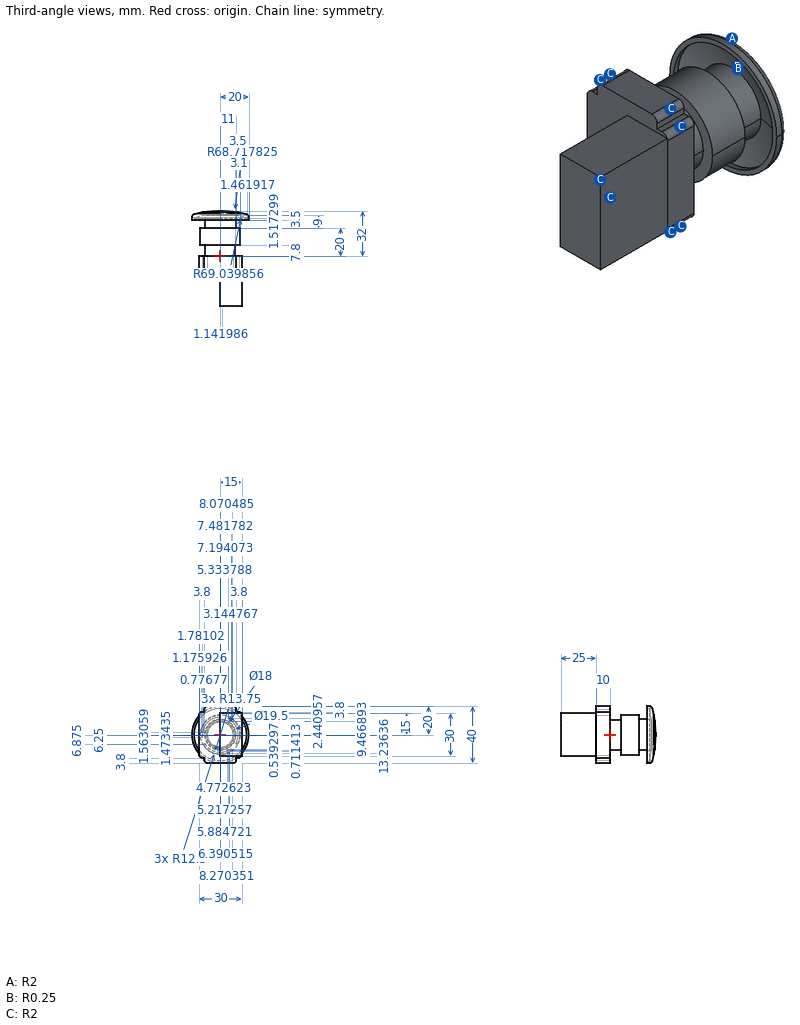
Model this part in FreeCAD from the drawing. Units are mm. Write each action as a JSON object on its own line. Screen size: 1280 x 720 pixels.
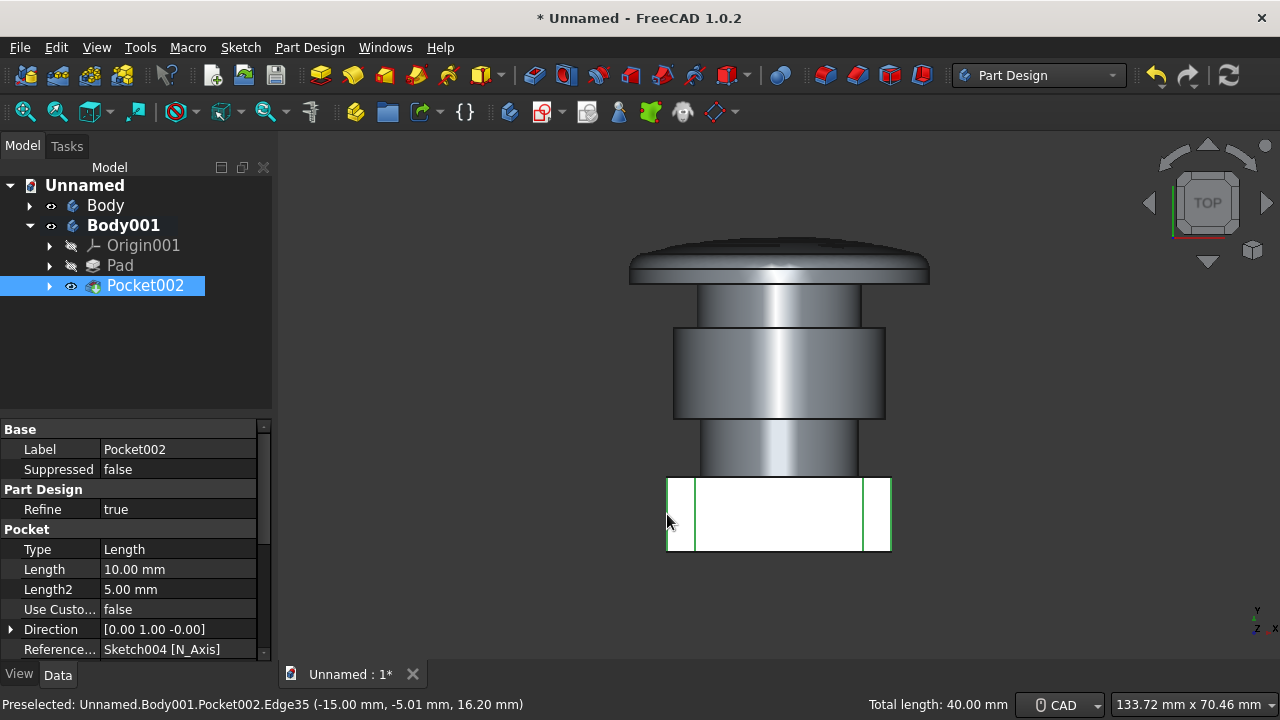
{"action": "key", "text": "0"}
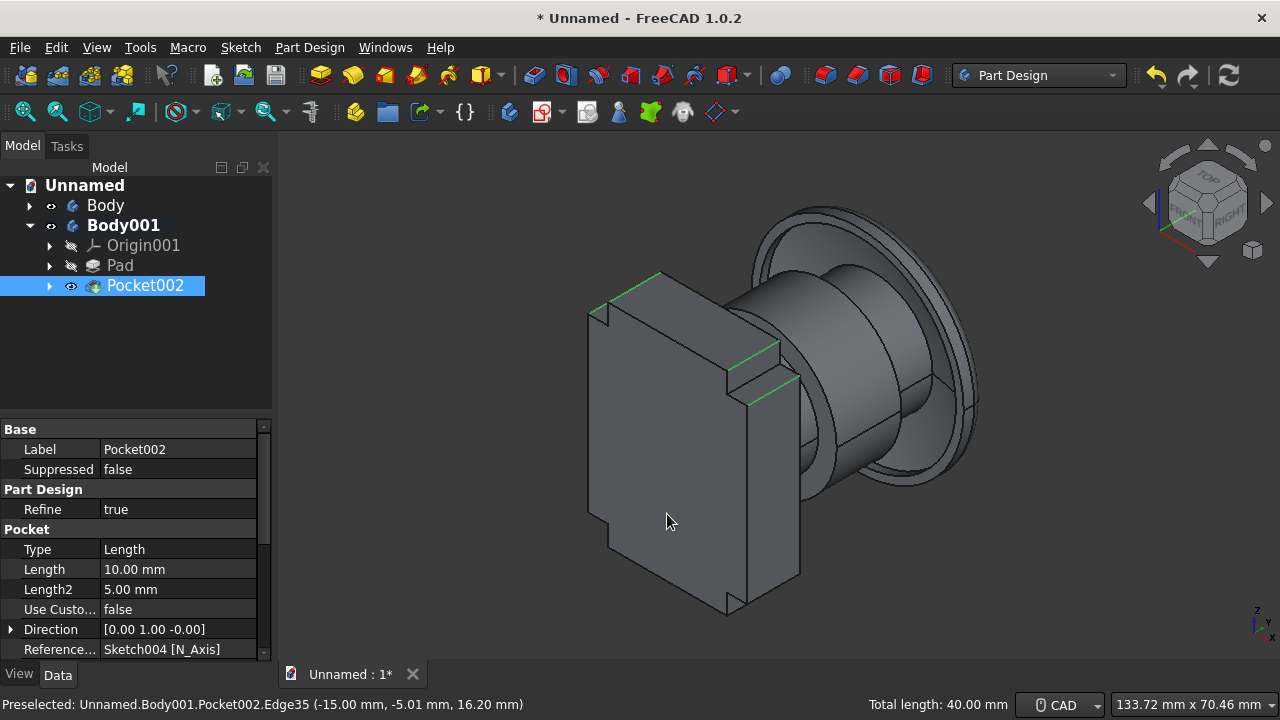
{"action": "key", "text": "1"}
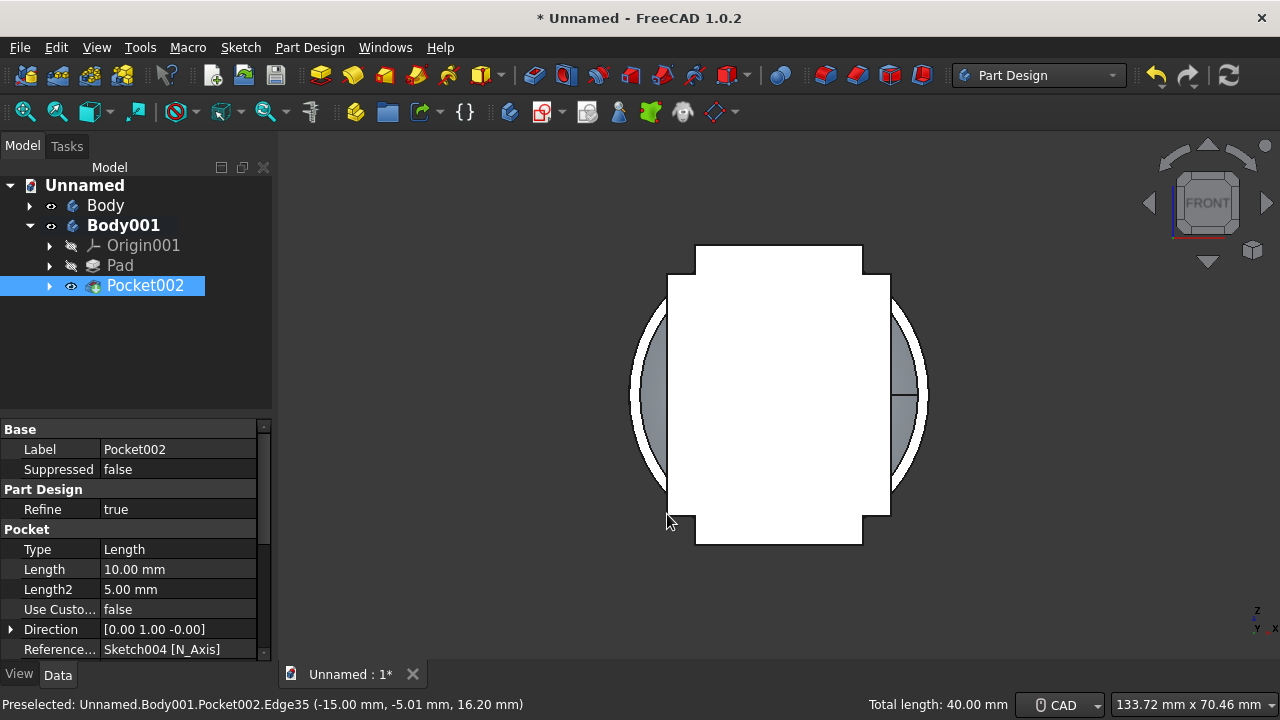
{"action": "key", "text": "3"}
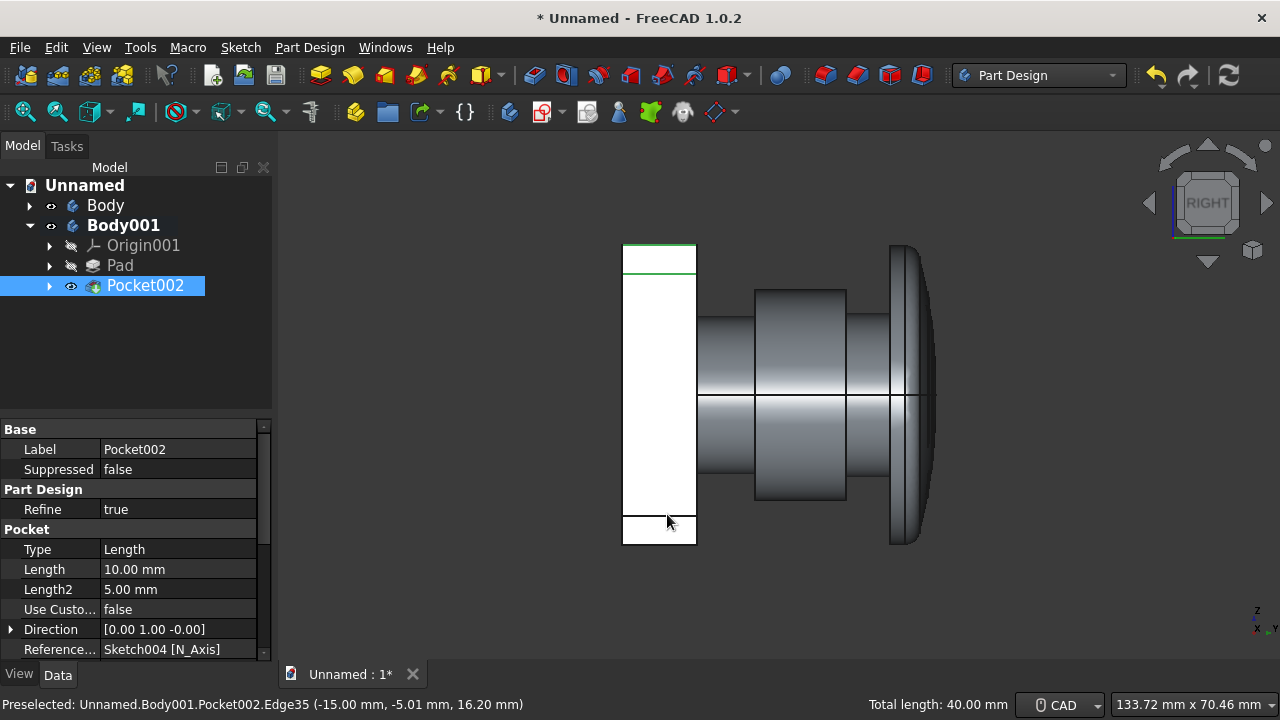
{"action": "left_click", "coordinate": [659, 544], "text": "ctrl"}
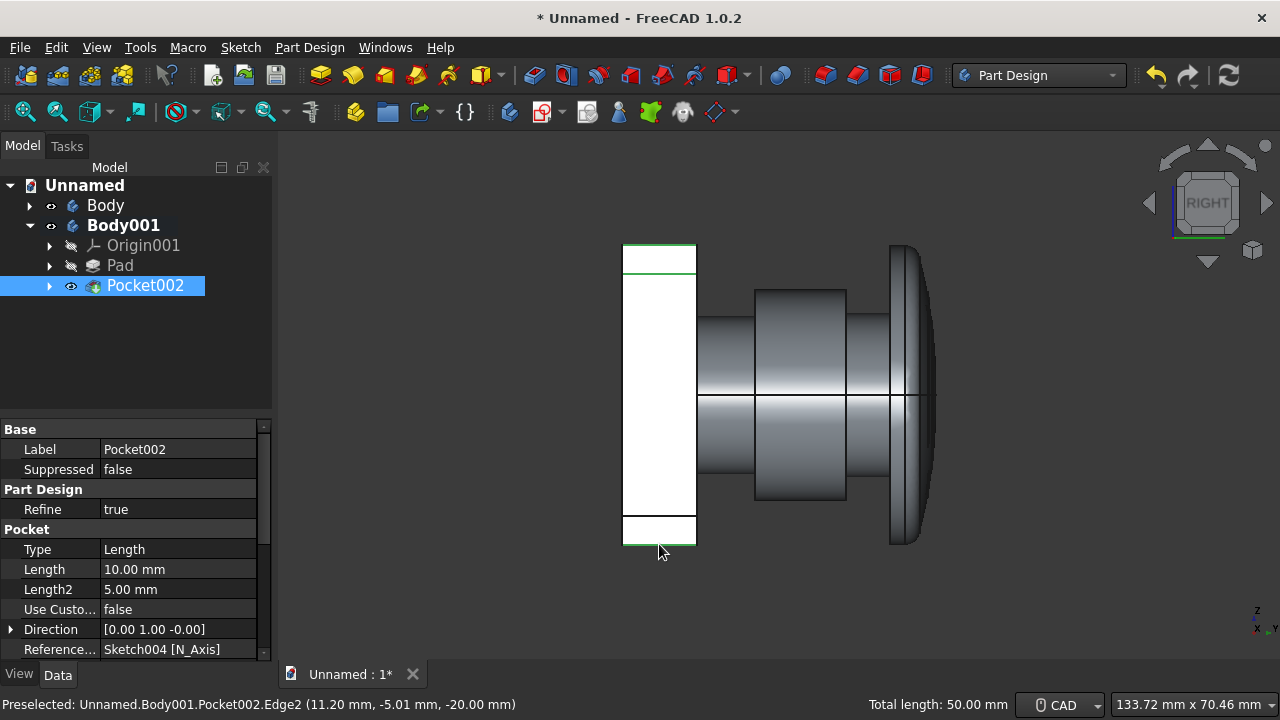
{"action": "left_click", "coordinate": [659, 515], "text": "ctrl"}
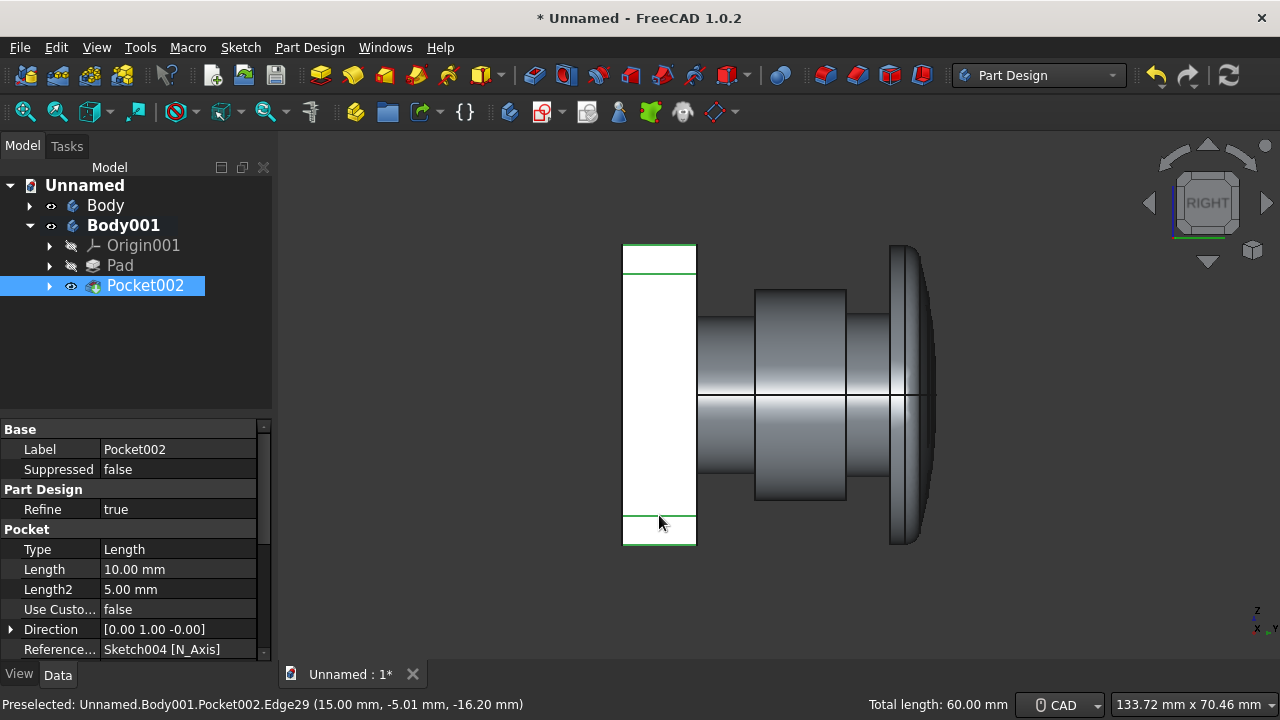
{"action": "key", "text": "5"}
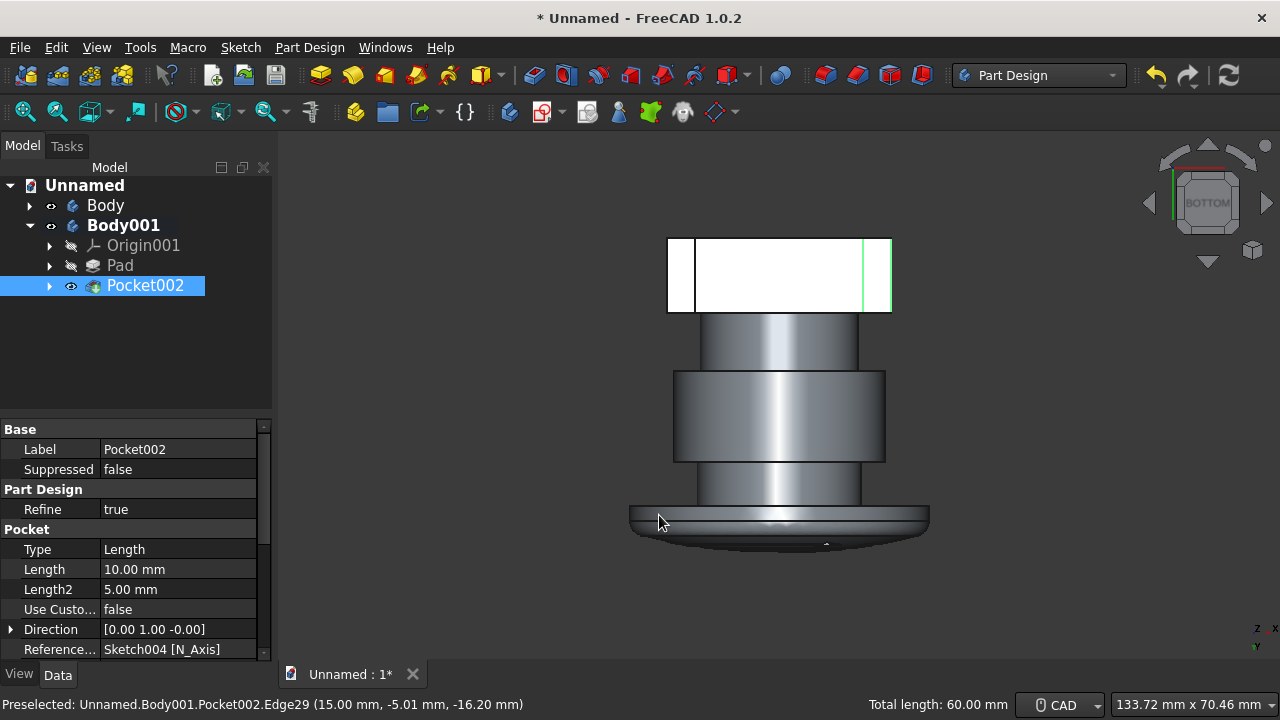
{"action": "left_click", "coordinate": [26, 112]}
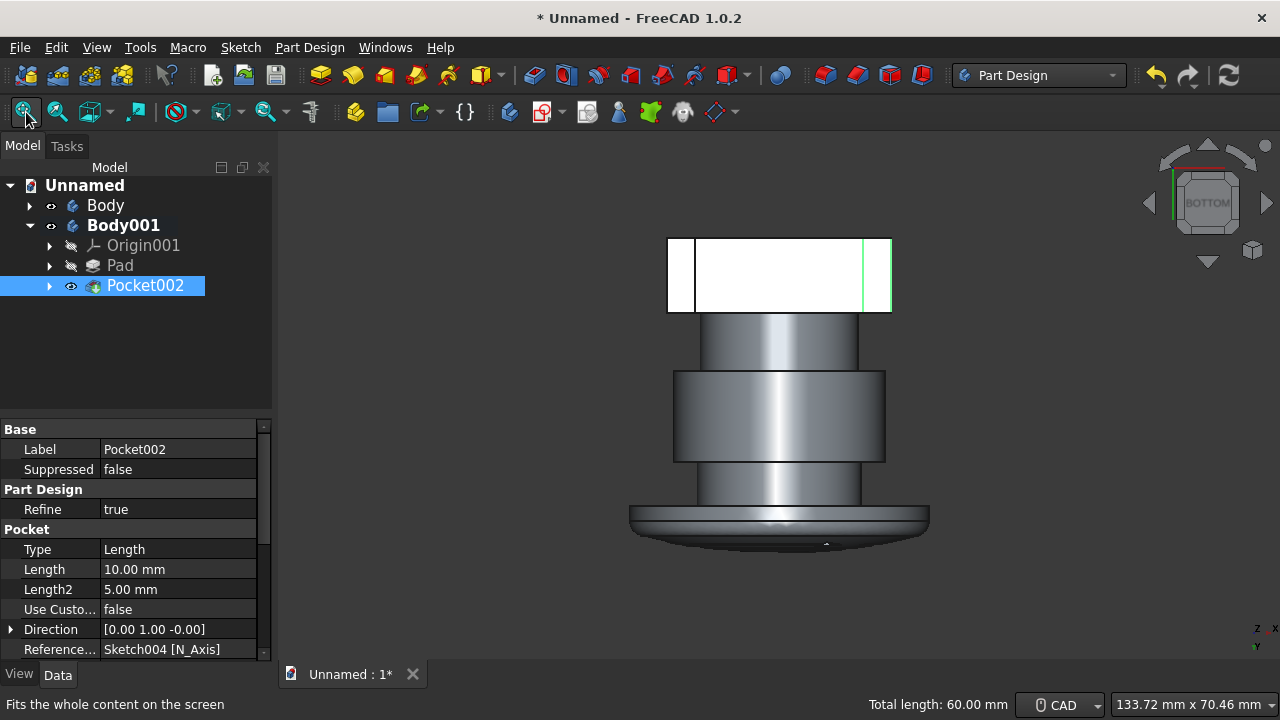
{"action": "left_click", "coordinate": [667, 274], "text": "ctrl"}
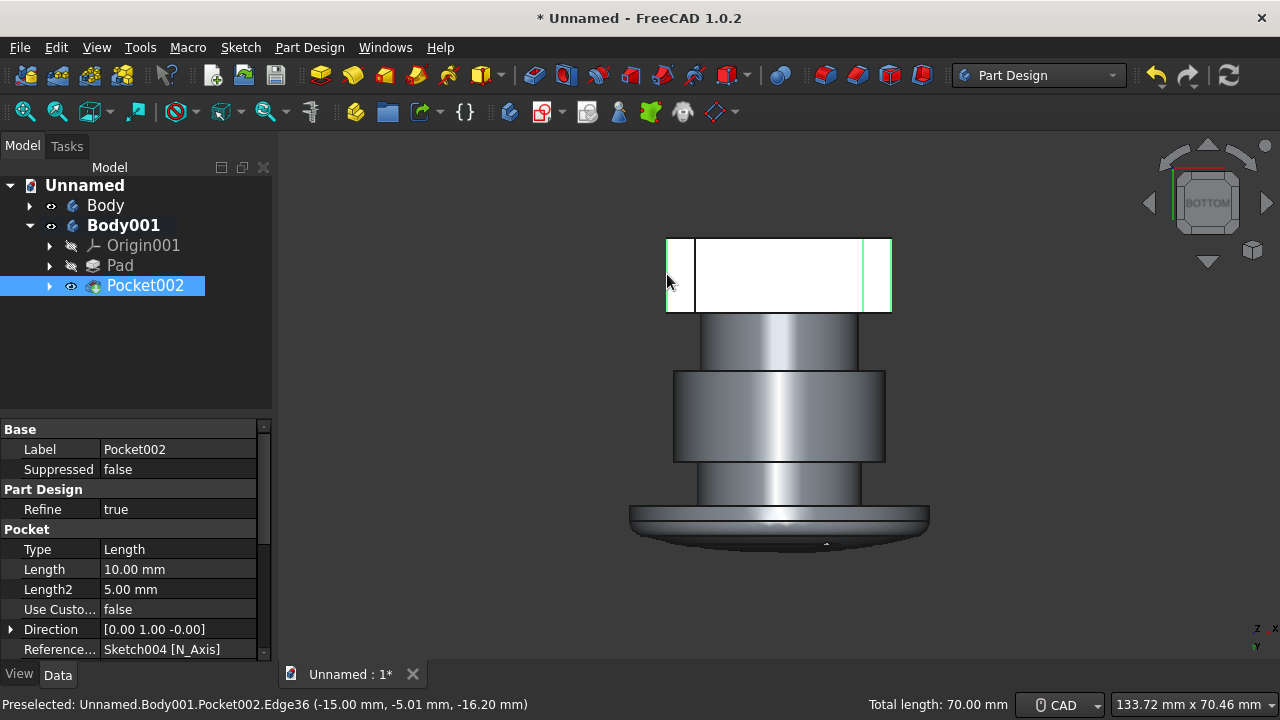
{"action": "left_click", "coordinate": [695, 274], "text": "ctrl"}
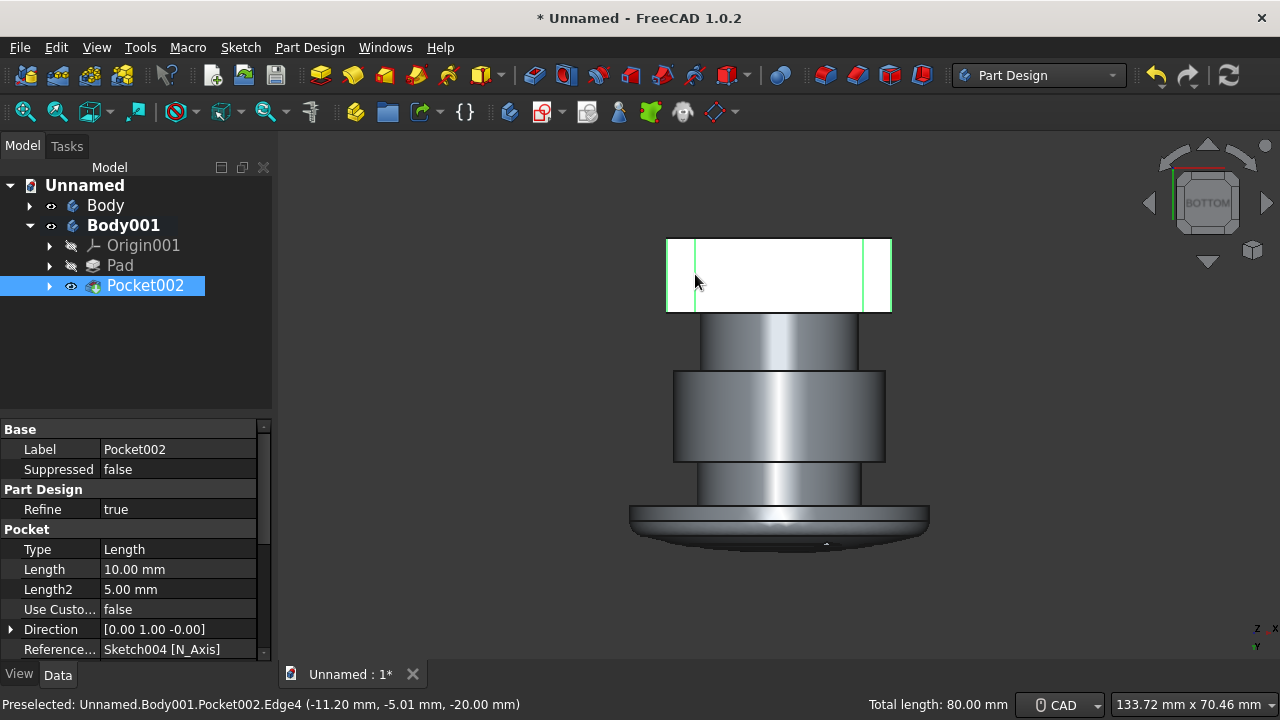
{"action": "left_click", "coordinate": [826, 76]}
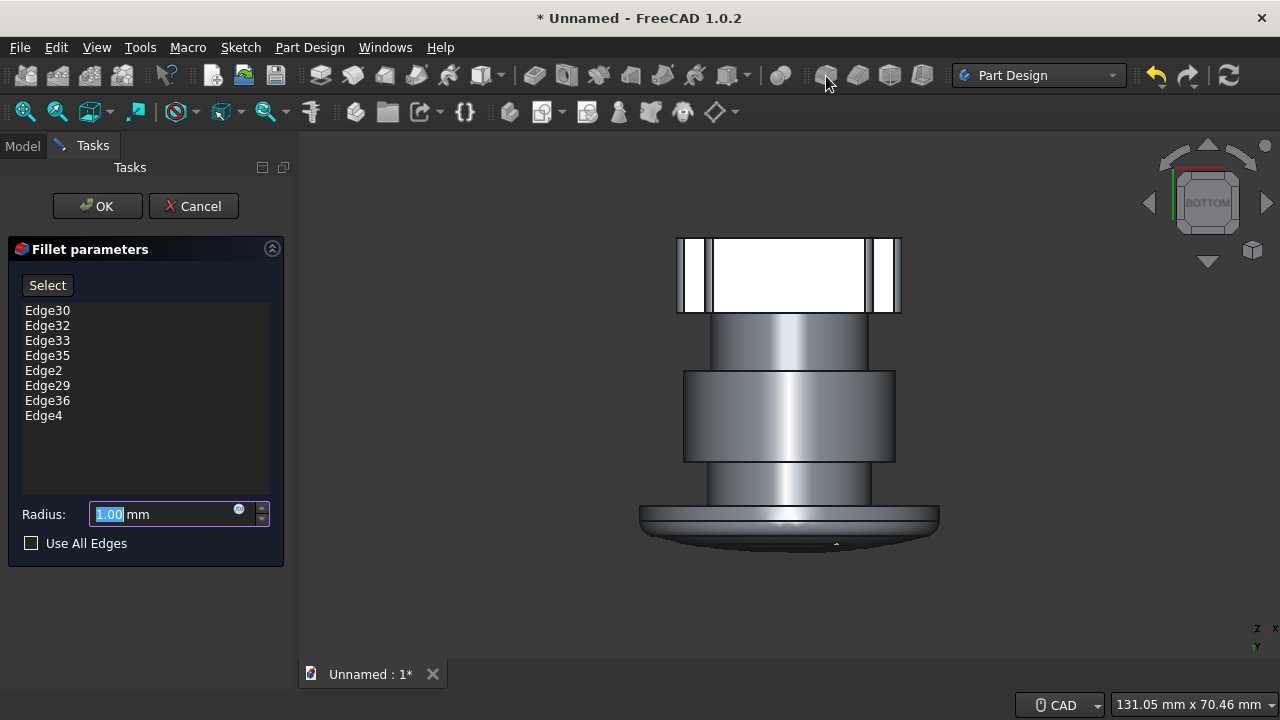
{"action": "type", "text": "2"}
{"action": "key", "text": "Tab"}